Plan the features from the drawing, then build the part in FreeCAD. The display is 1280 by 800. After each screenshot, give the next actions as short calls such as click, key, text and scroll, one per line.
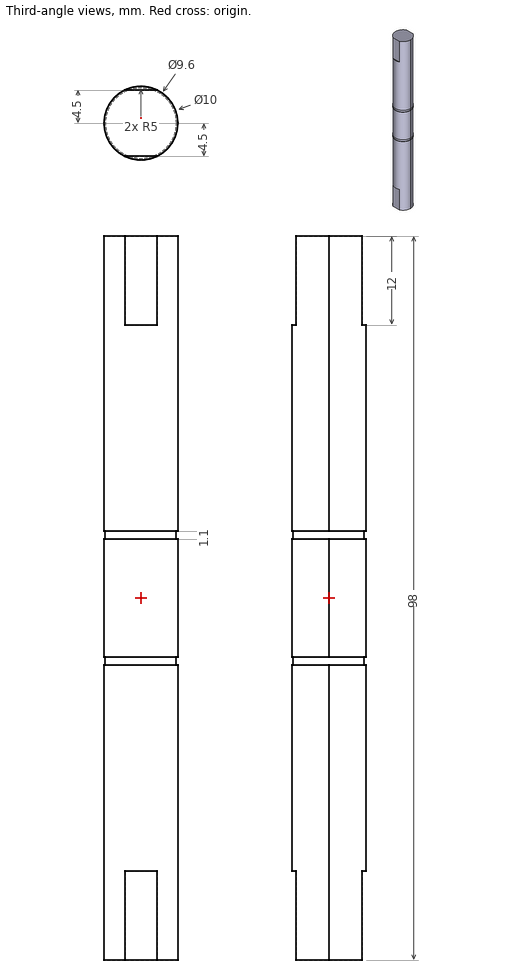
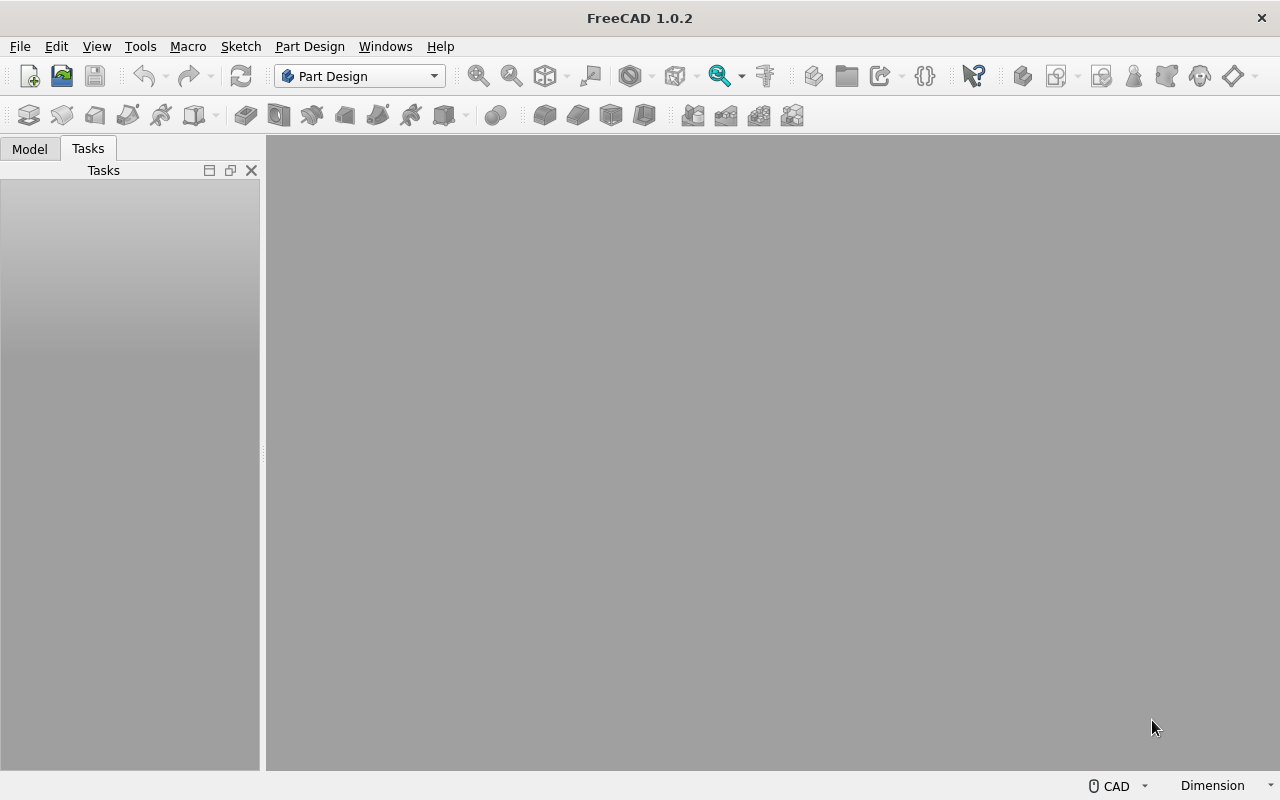
click(29, 76)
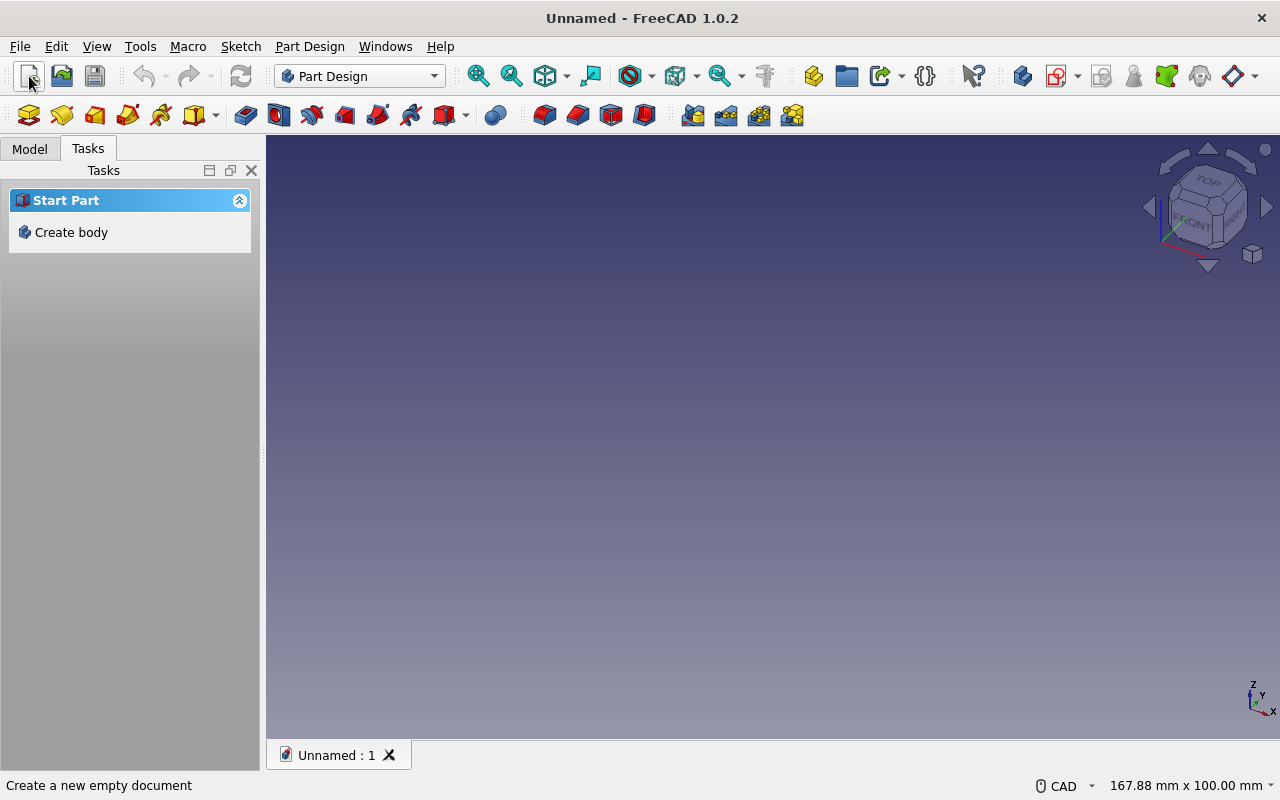
click(1056, 76)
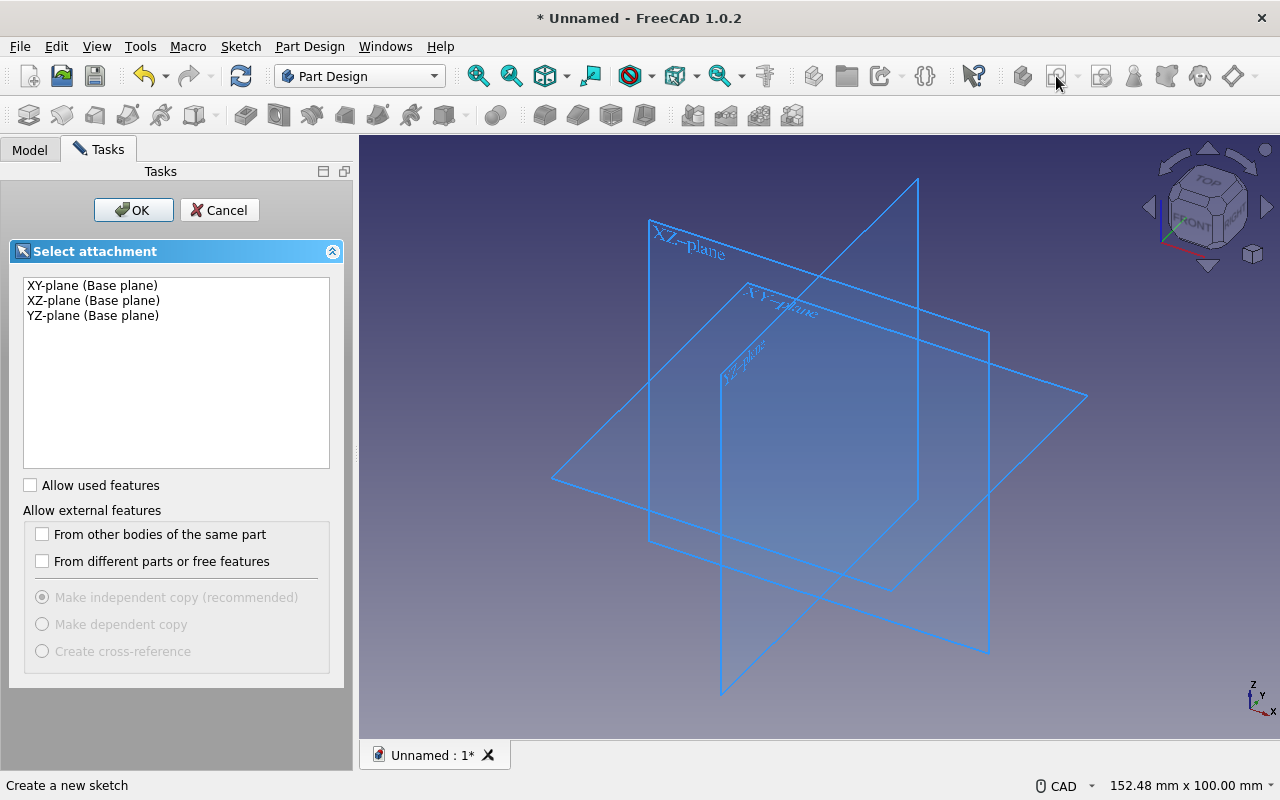
click(84, 286)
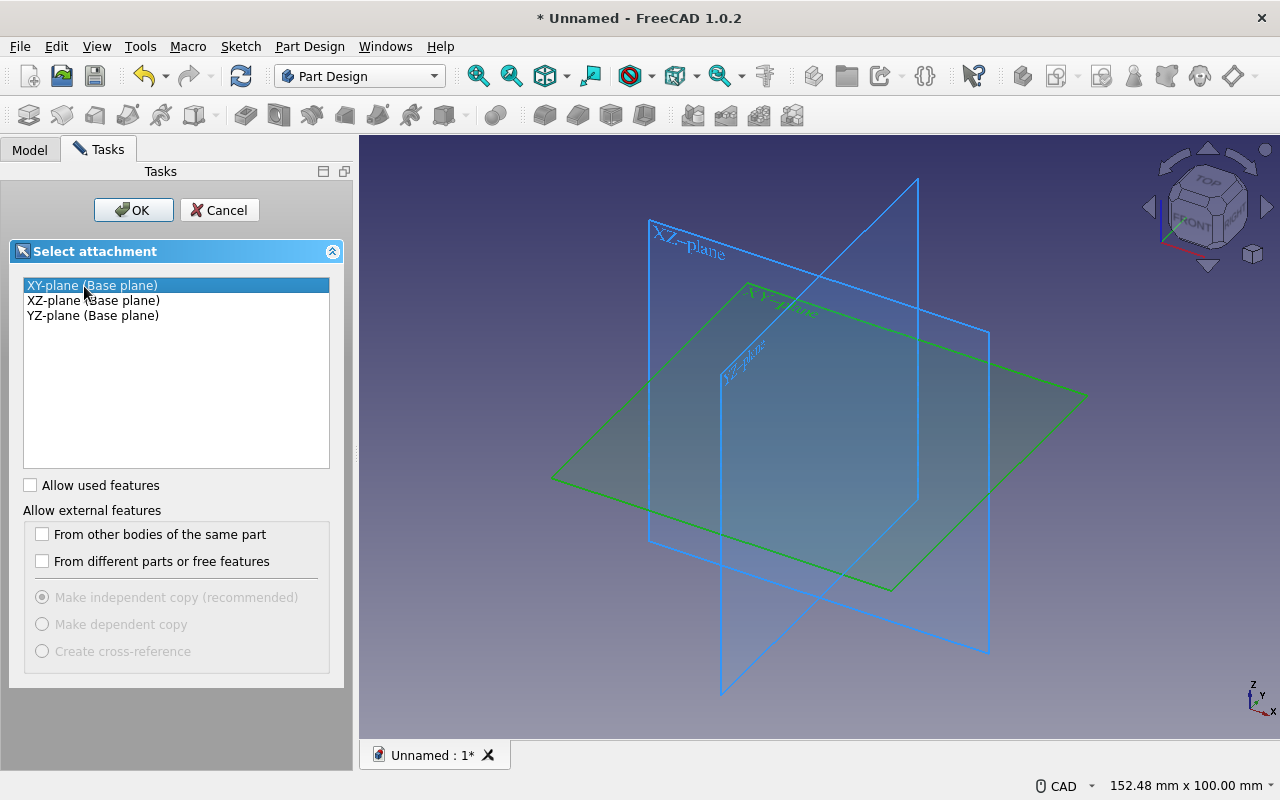
click(134, 210)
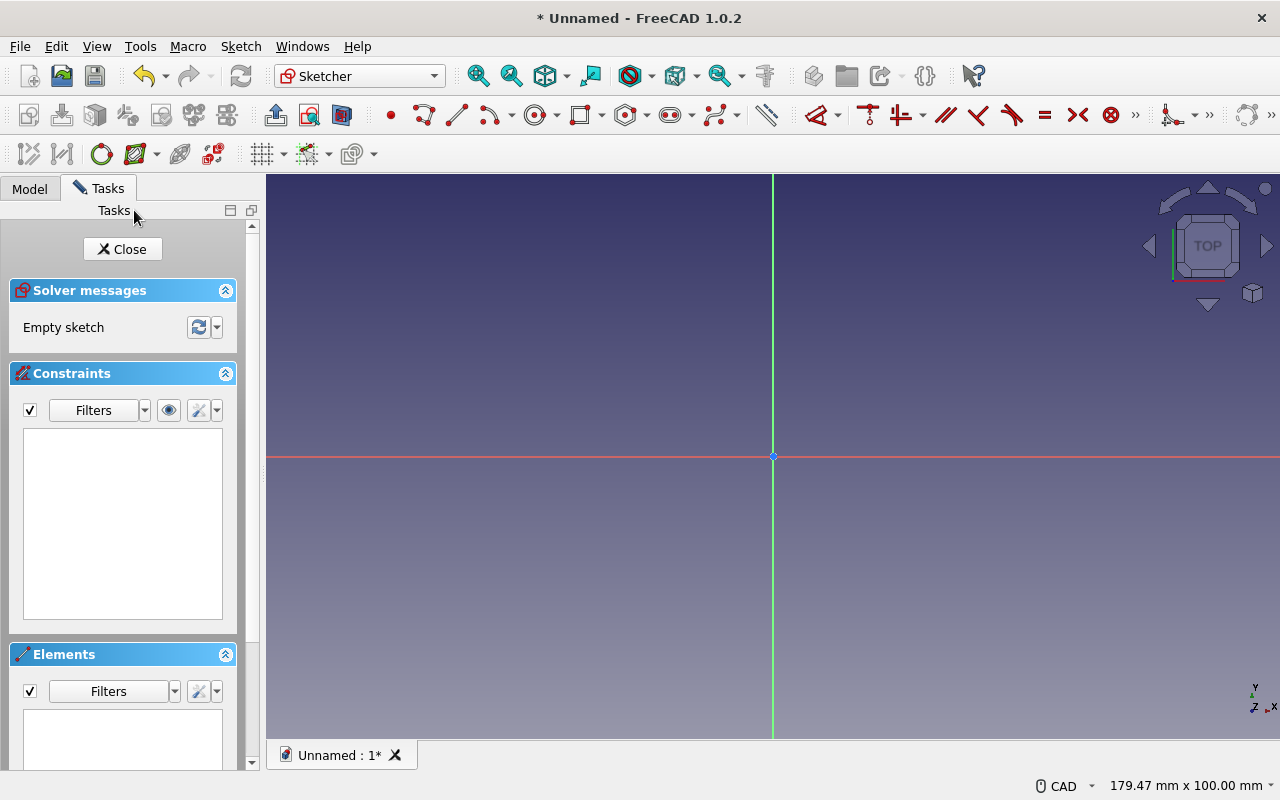
scroll(787, 456, up, 9)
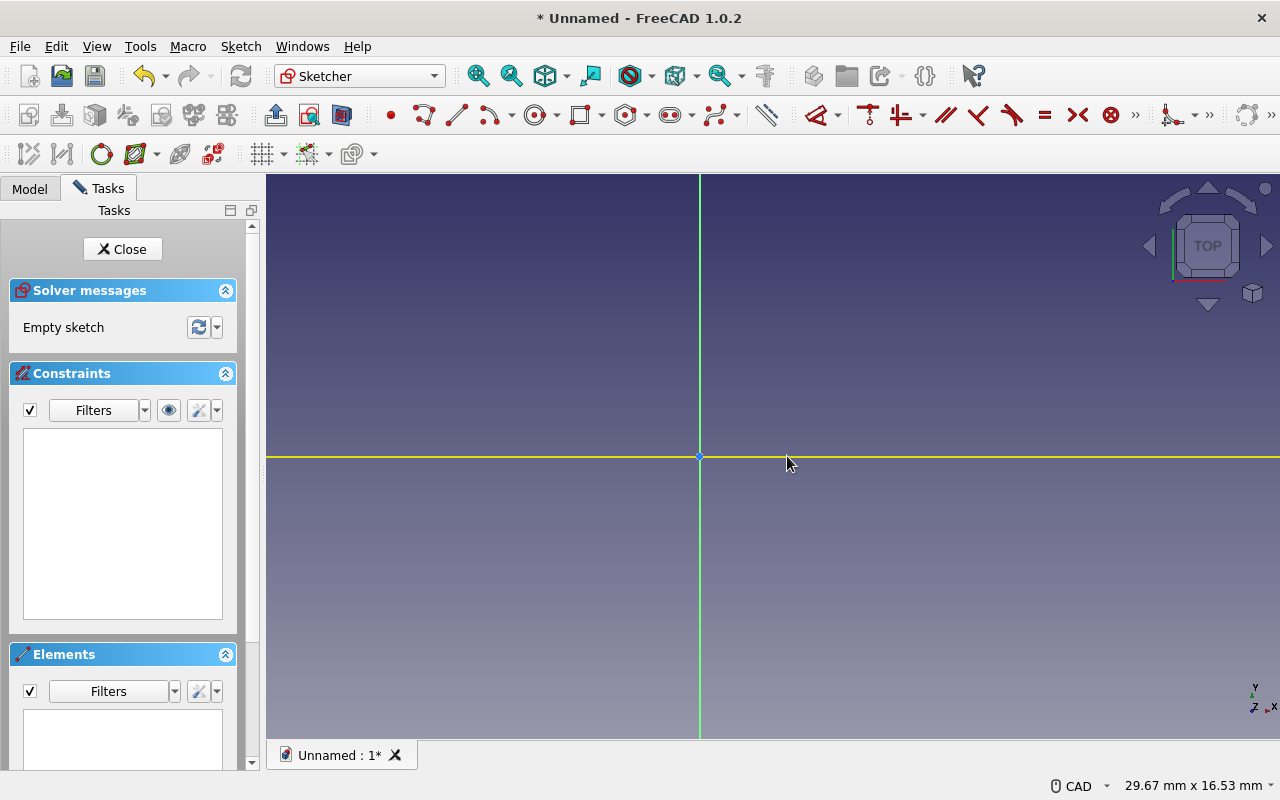
click(534, 116)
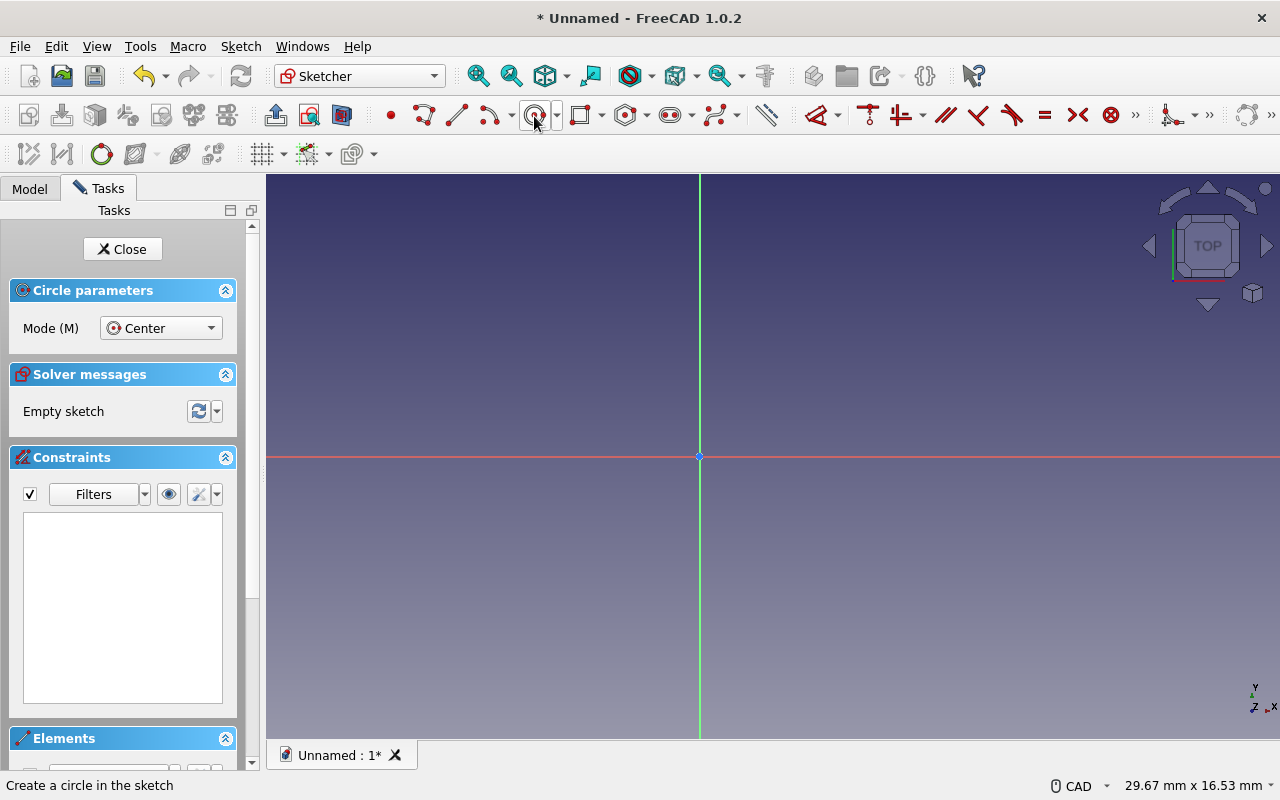
click(700, 456)
click(821, 336)
key(Escape)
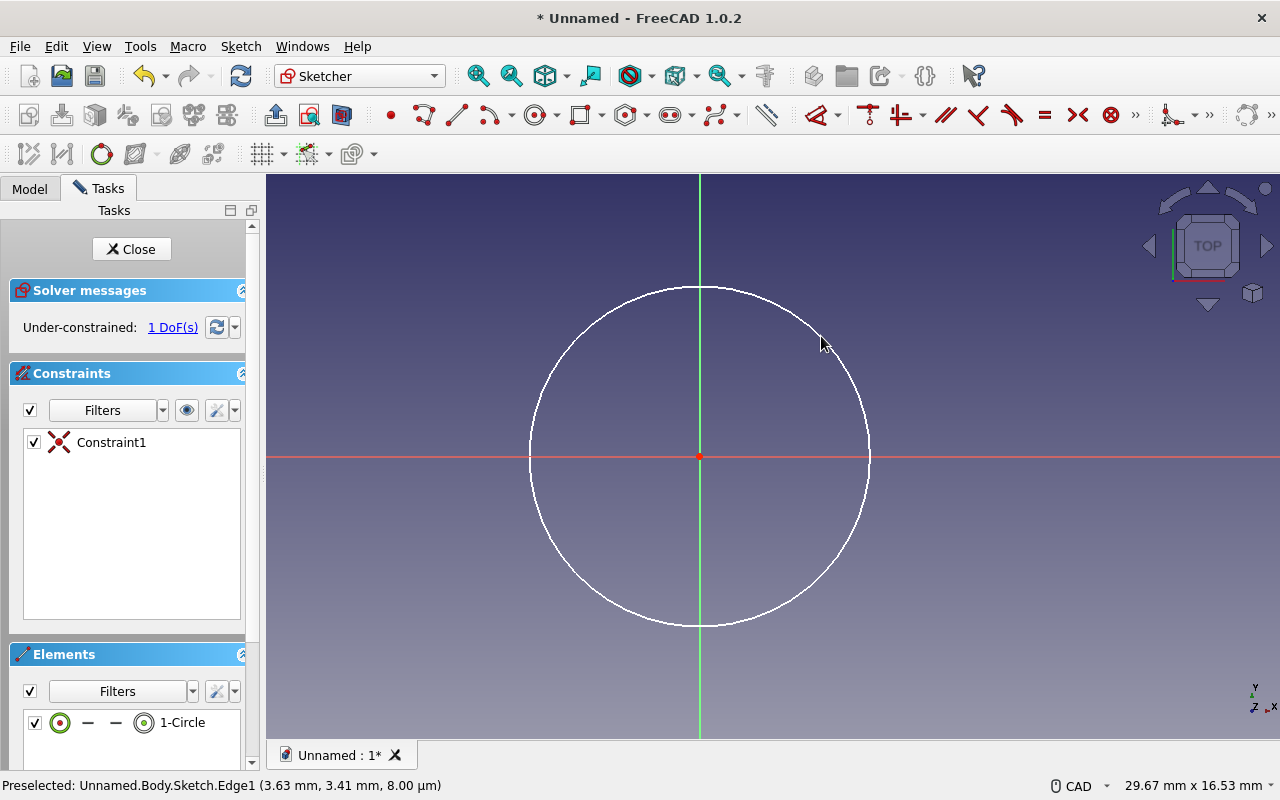
click(816, 116)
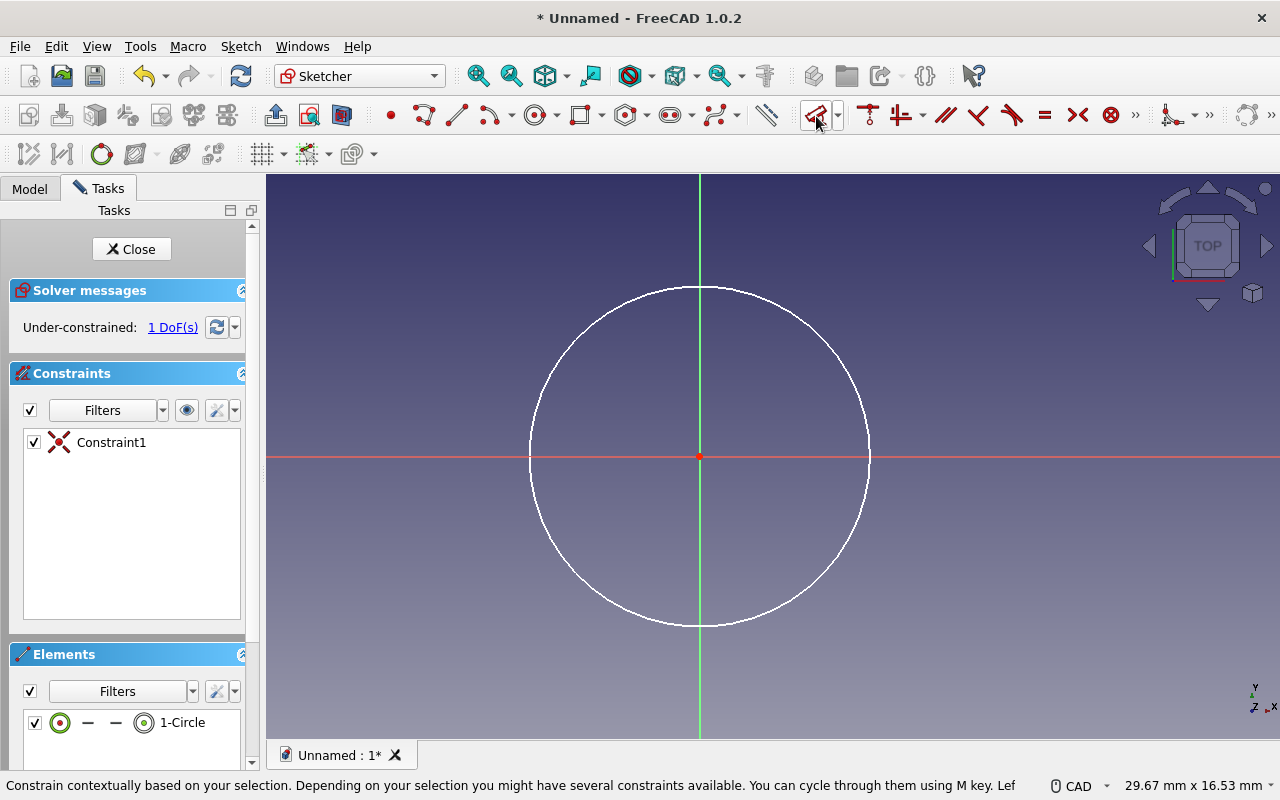
click(820, 336)
click(843, 313)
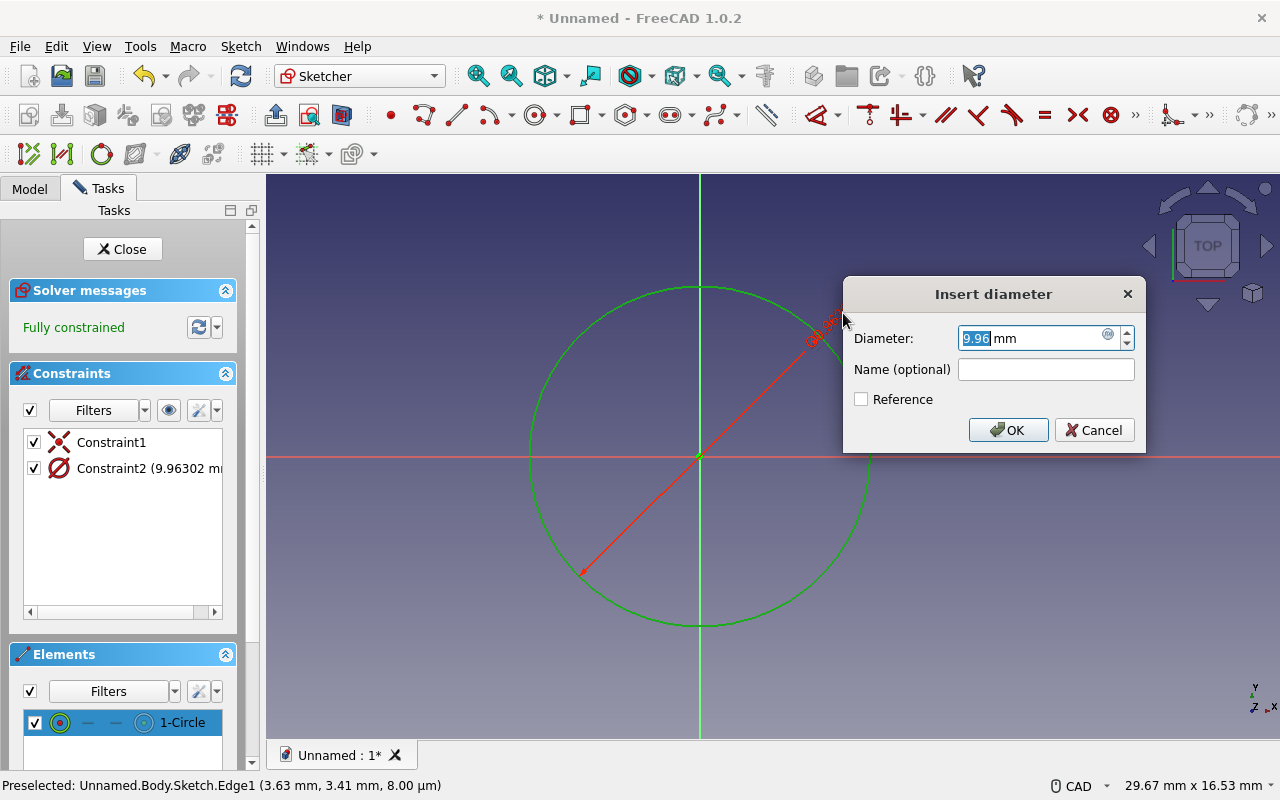
text(10)
key(Return)
key(Escape)